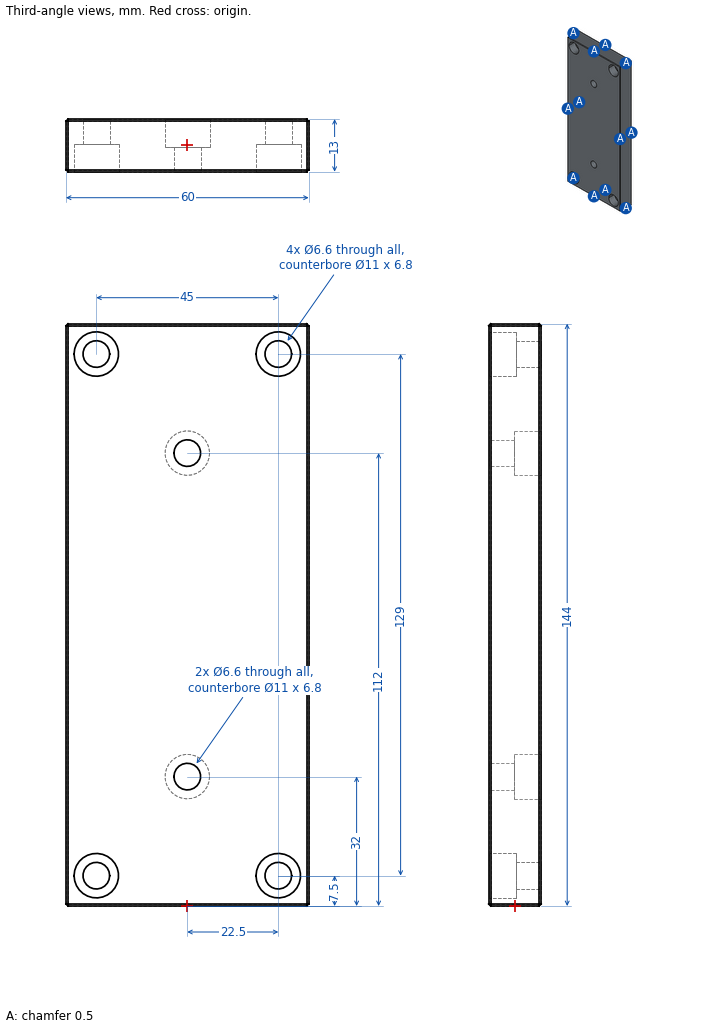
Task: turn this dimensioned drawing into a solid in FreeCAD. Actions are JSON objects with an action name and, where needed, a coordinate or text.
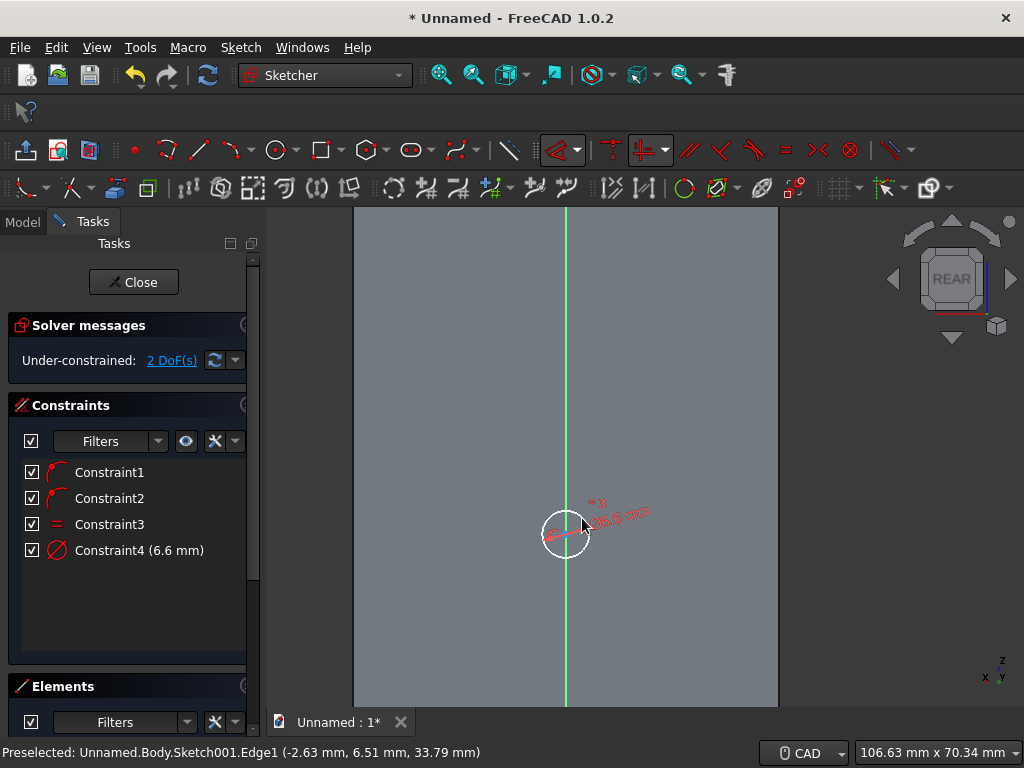
{"action": "left_click", "coordinate": [566, 534]}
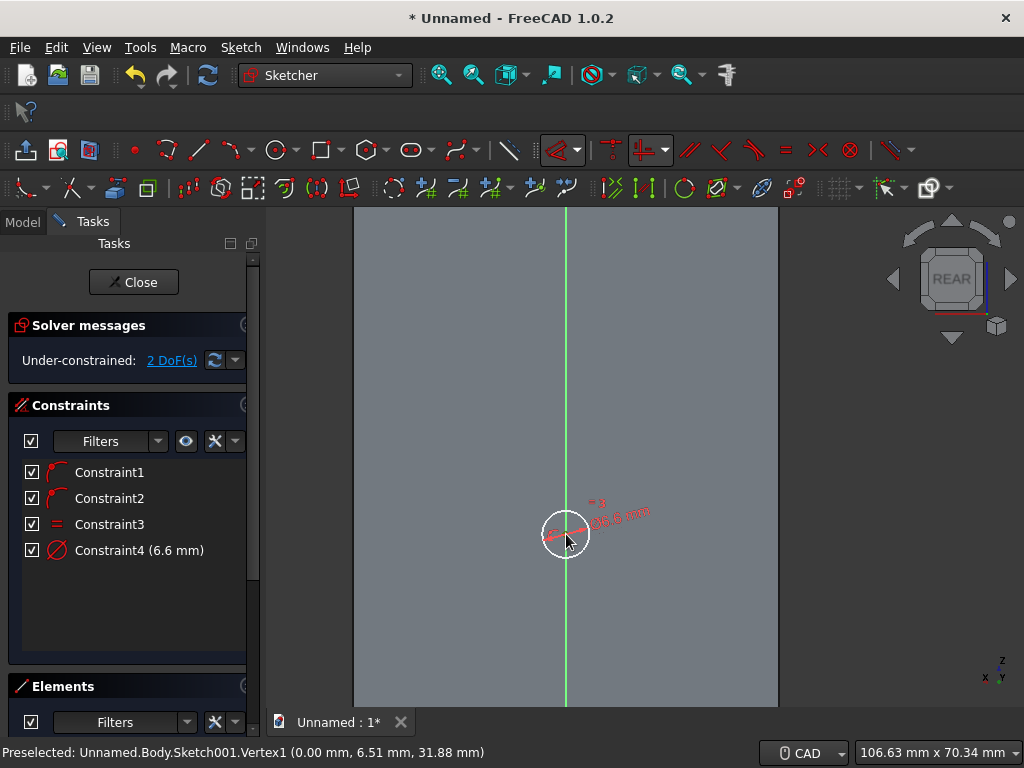
{"action": "key", "text": "i"}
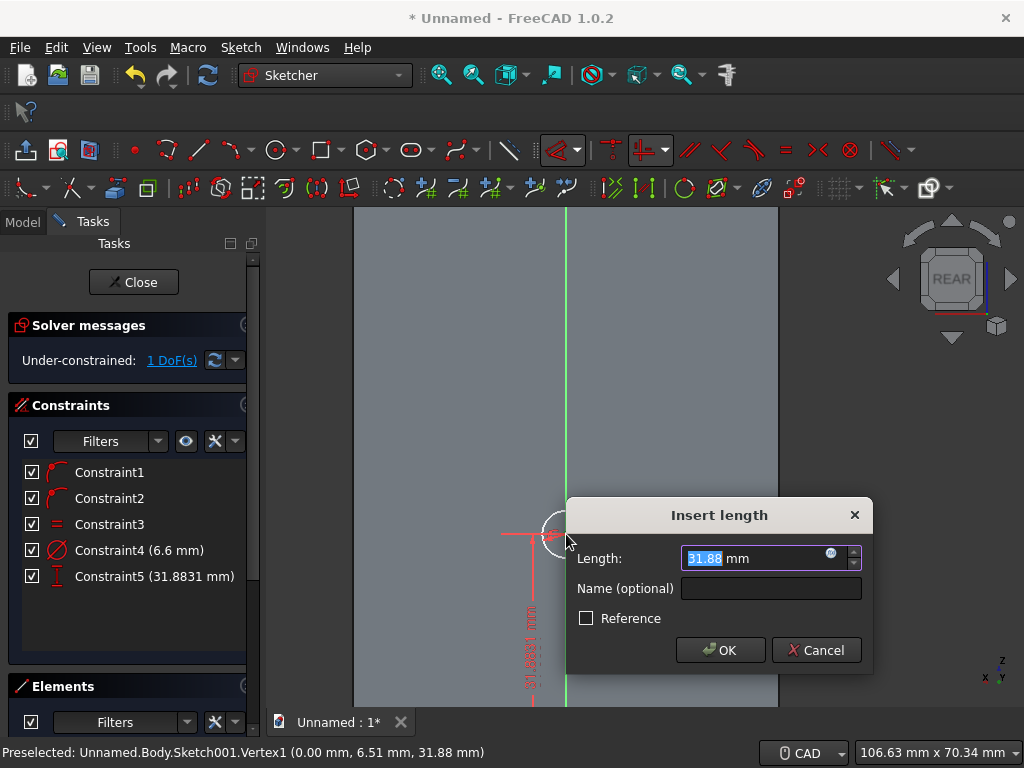
{"action": "type", "text": "32"}
{"action": "key", "text": "Return"}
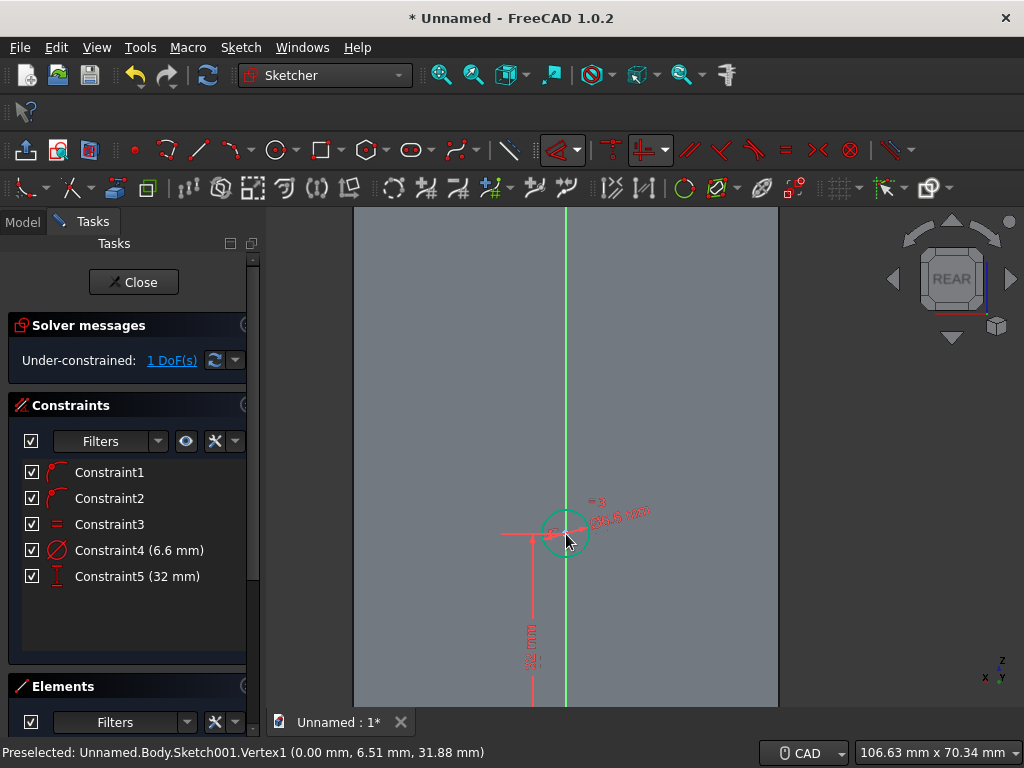
{"action": "scroll", "coordinate": [583, 519], "scroll_direction": "down", "scroll_amount": 5}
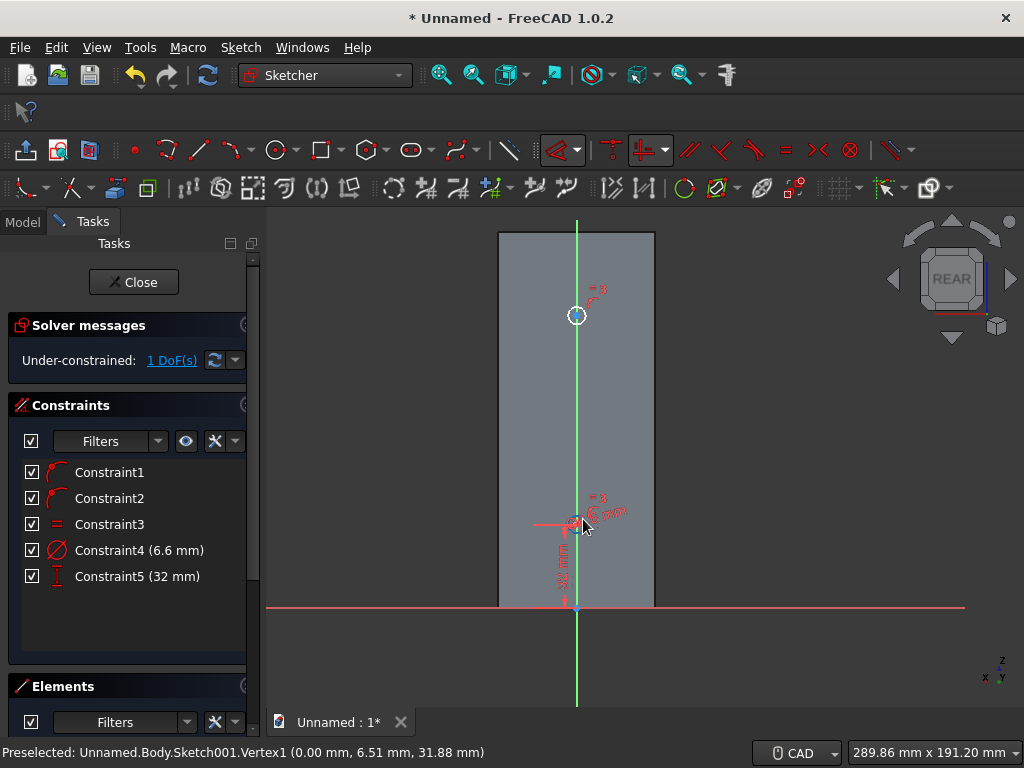
{"action": "left_click", "coordinate": [577, 316]}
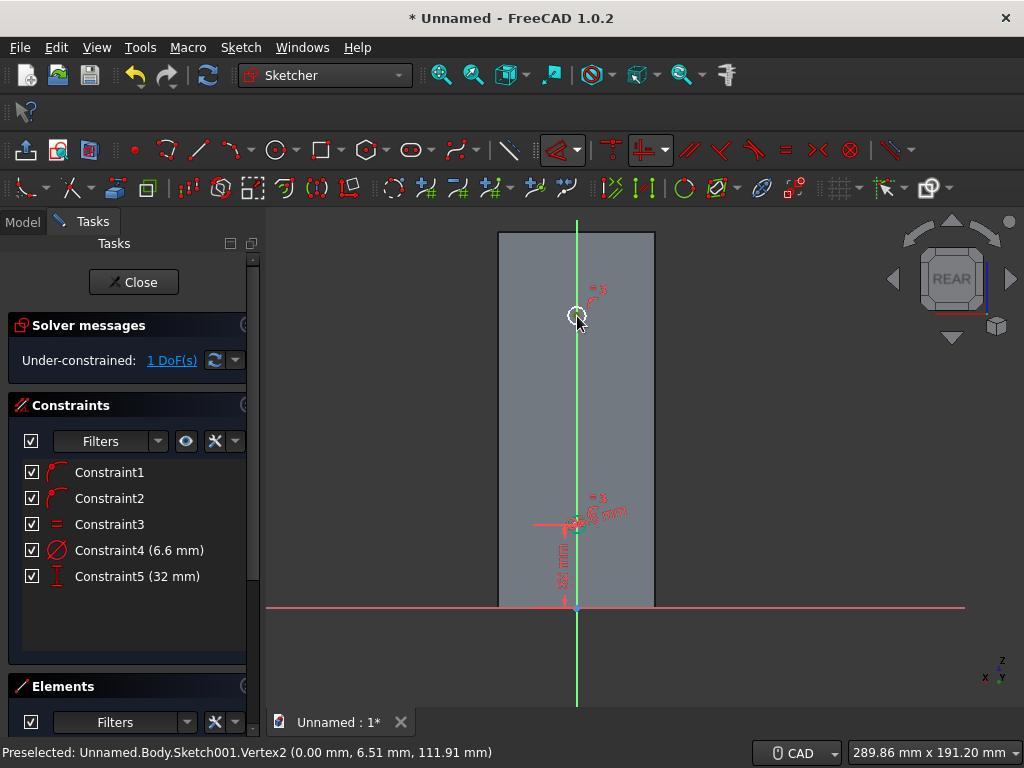
{"action": "key", "text": "i"}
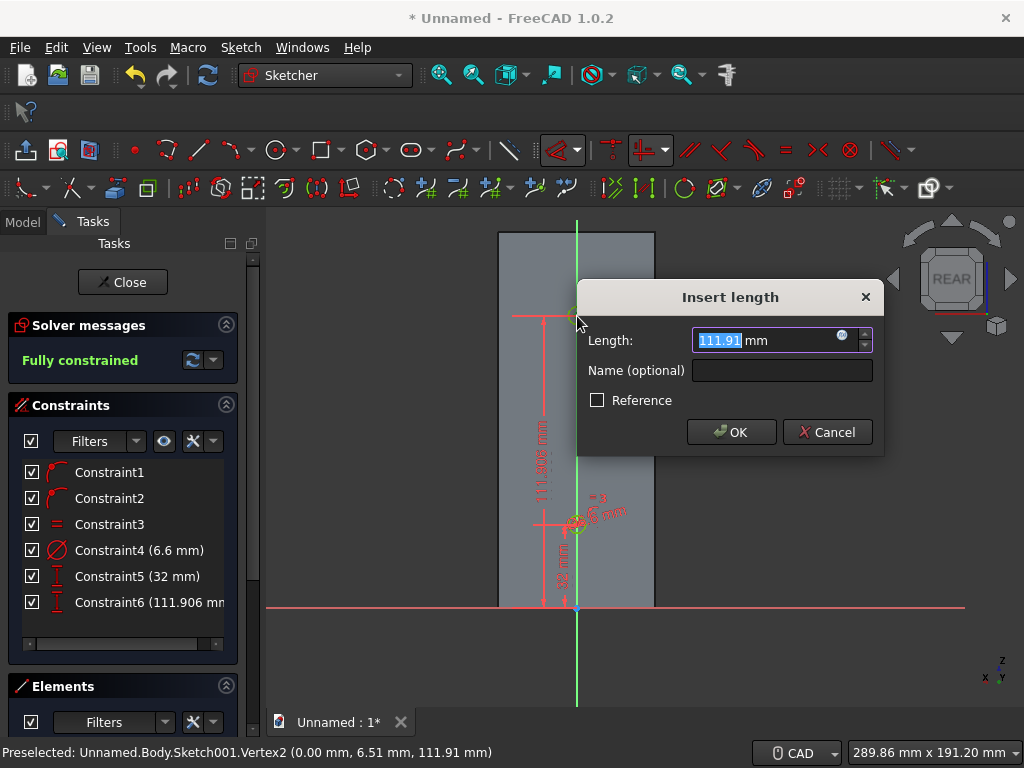
{"action": "type", "text": "112"}
{"action": "key", "text": "Return"}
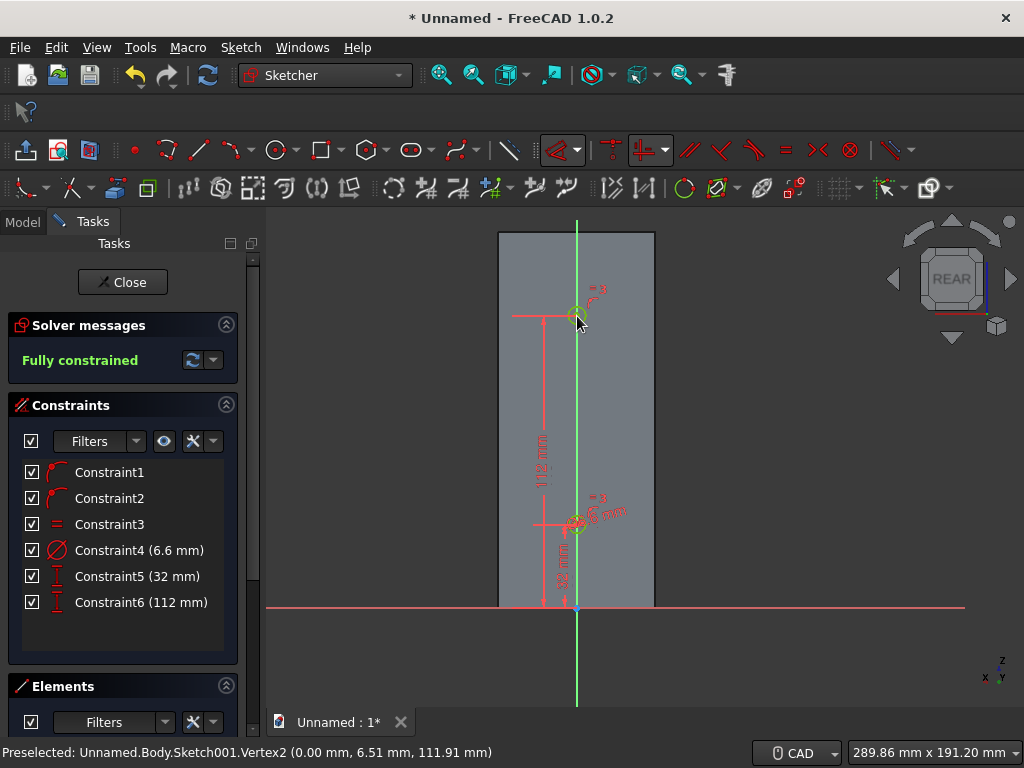
{"action": "left_click", "coordinate": [123, 282]}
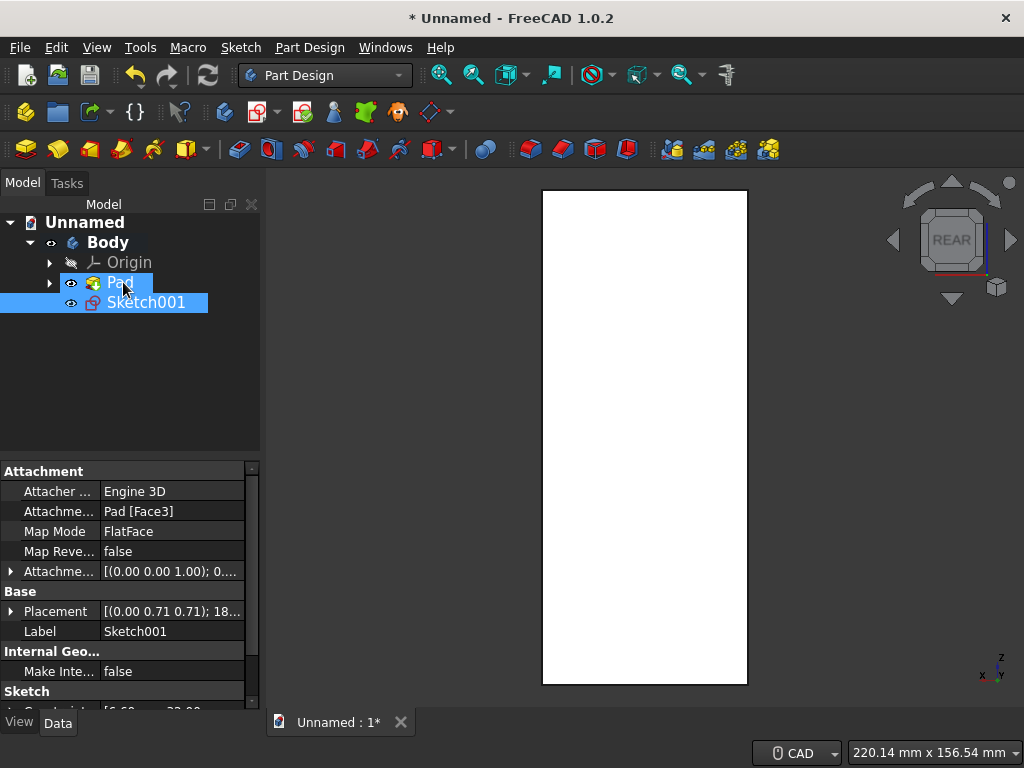
{"action": "left_click", "coordinate": [272, 150]}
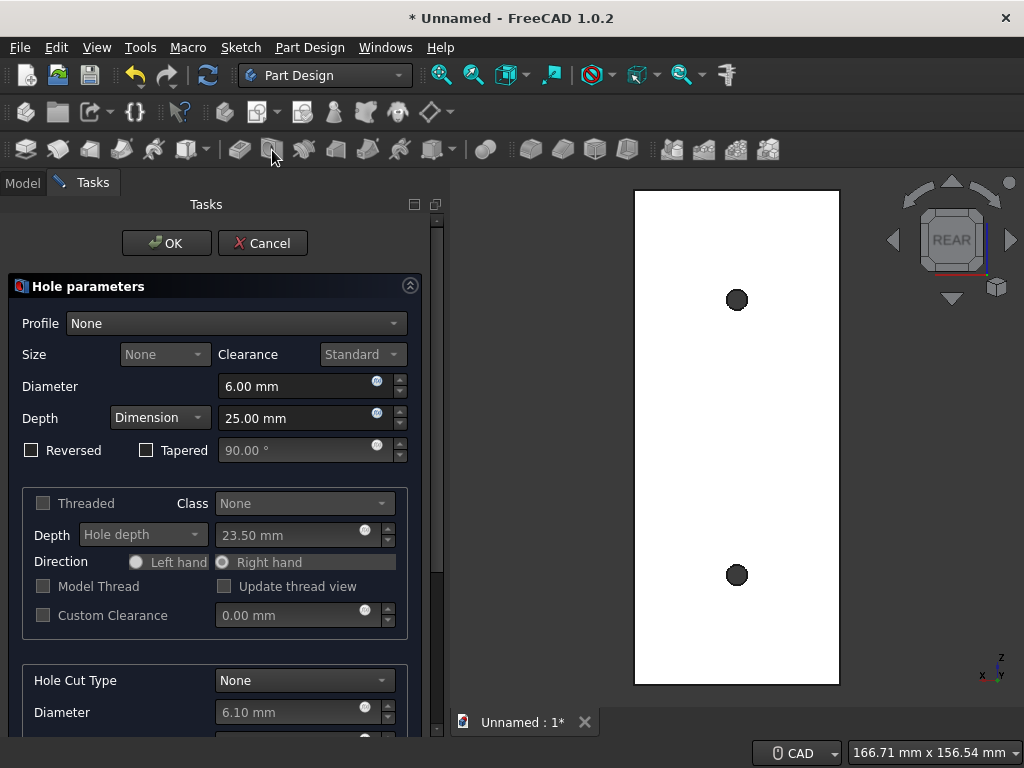
{"action": "triple_click", "coordinate": [305, 386]}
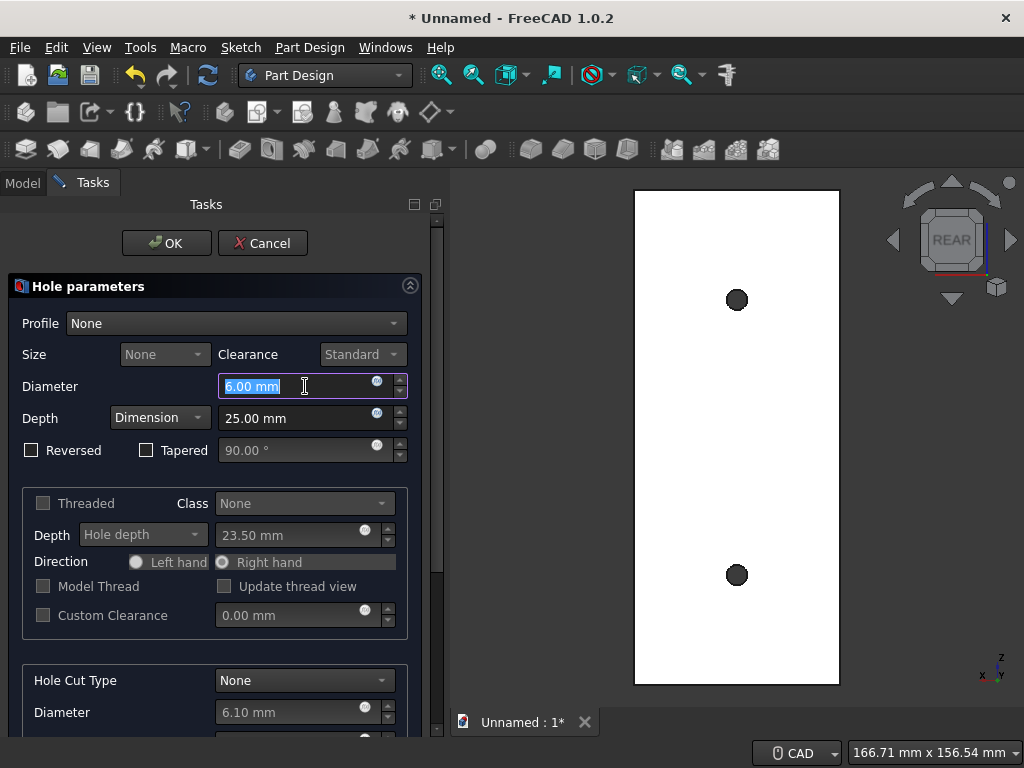
{"action": "type", "text": "6.6"}
{"action": "key", "text": "Tab"}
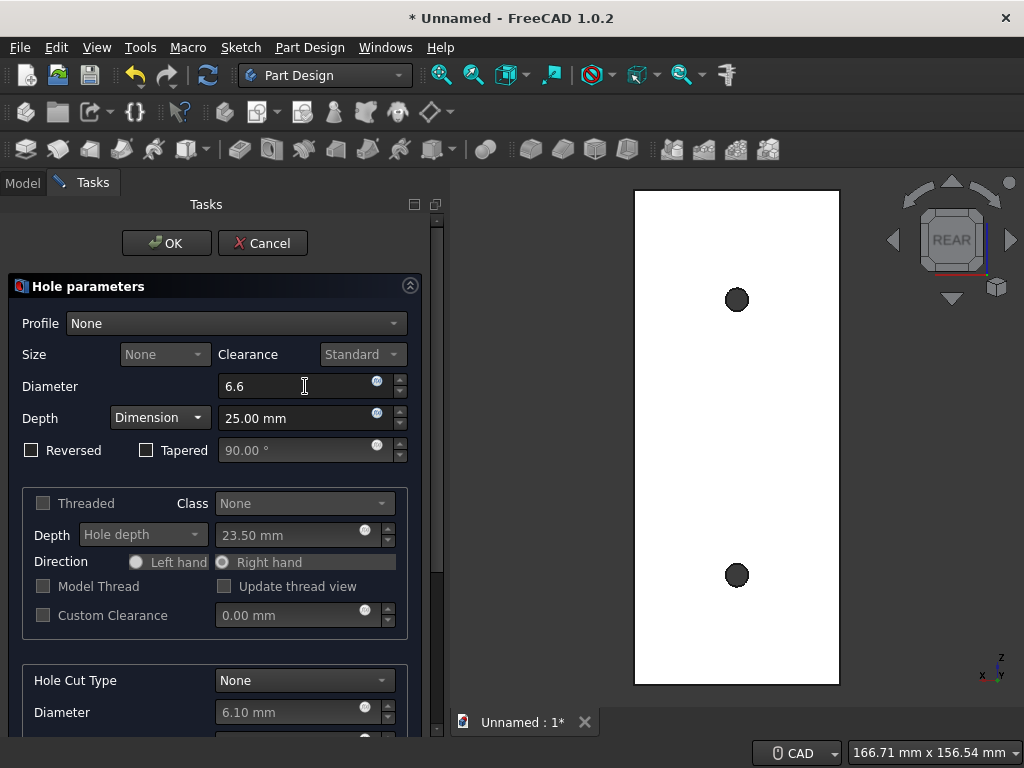
{"action": "left_click", "coordinate": [161, 418]}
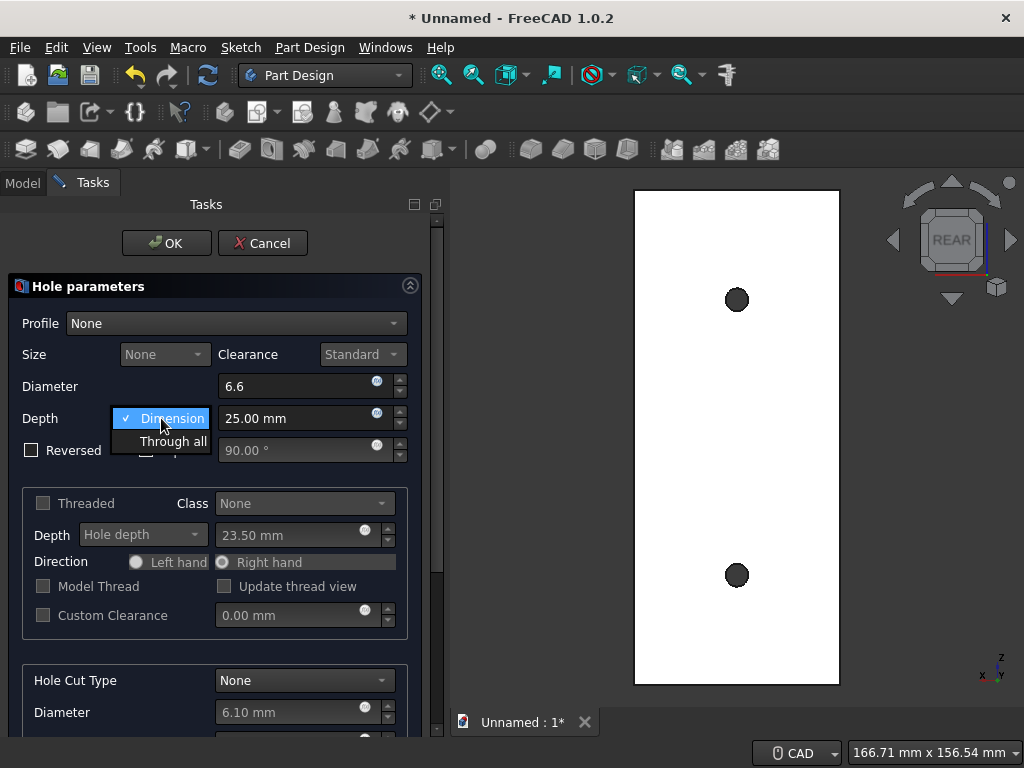
{"action": "left_click", "coordinate": [160, 442]}